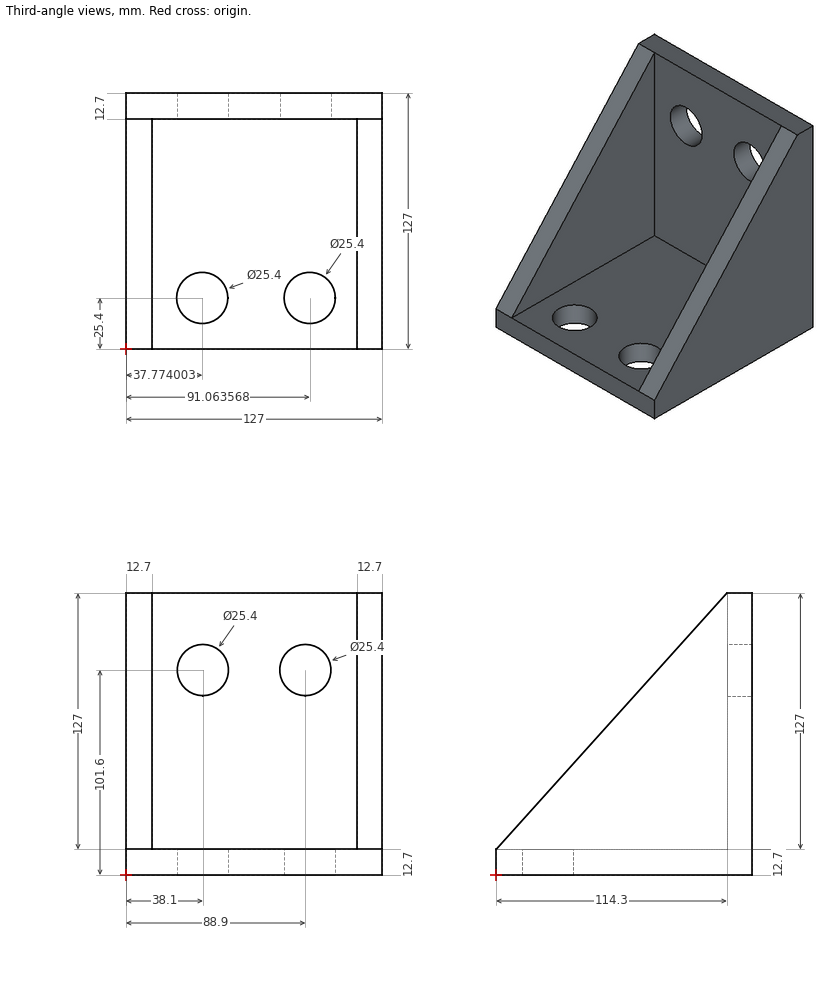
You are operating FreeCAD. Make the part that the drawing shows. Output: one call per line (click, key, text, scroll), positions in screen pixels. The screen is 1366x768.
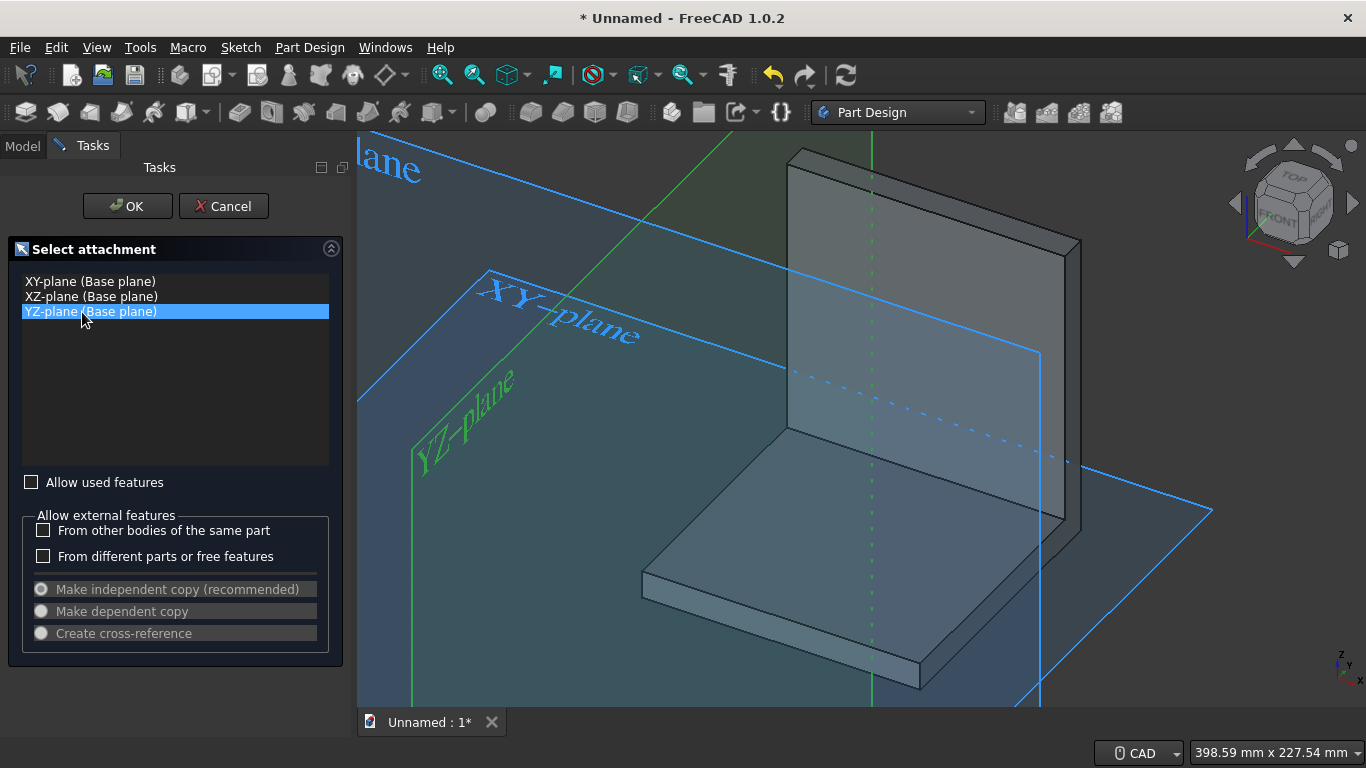
click(128, 206)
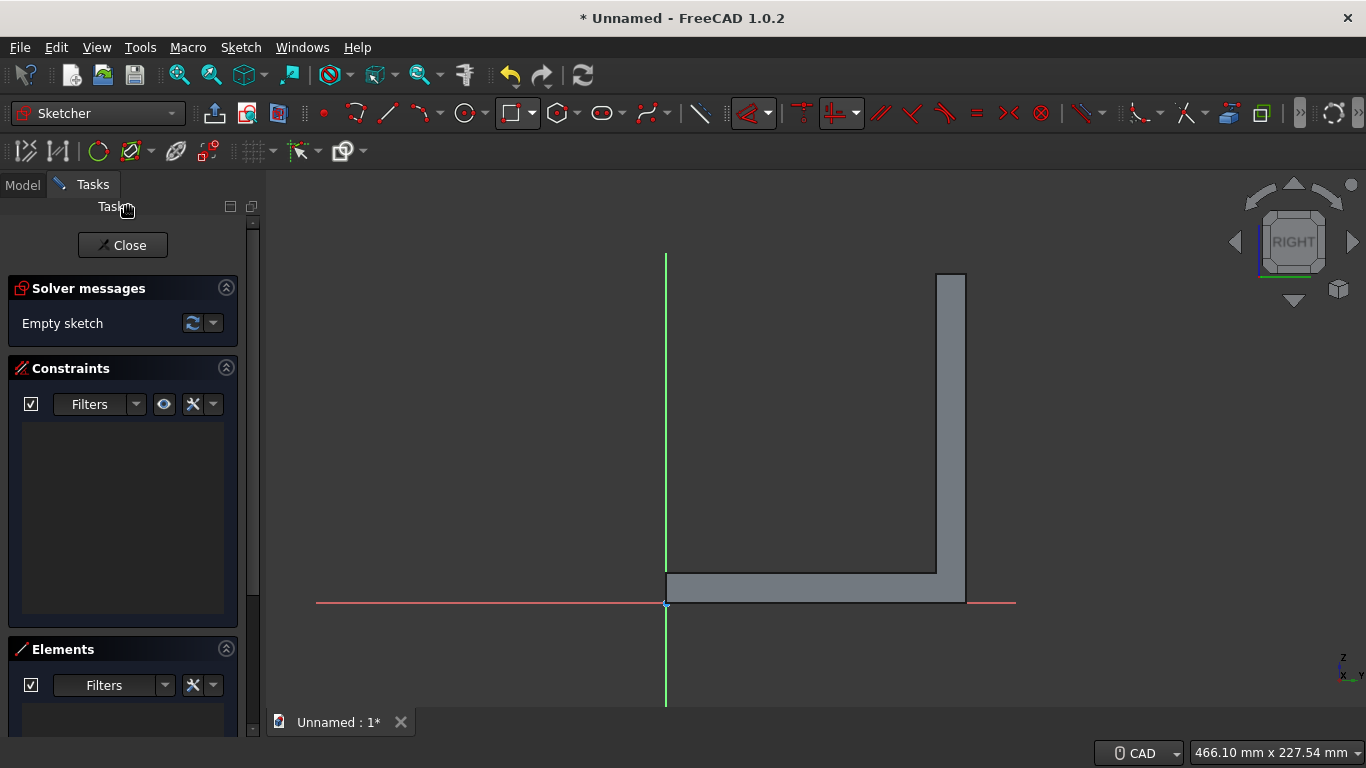
key(q)
key(s)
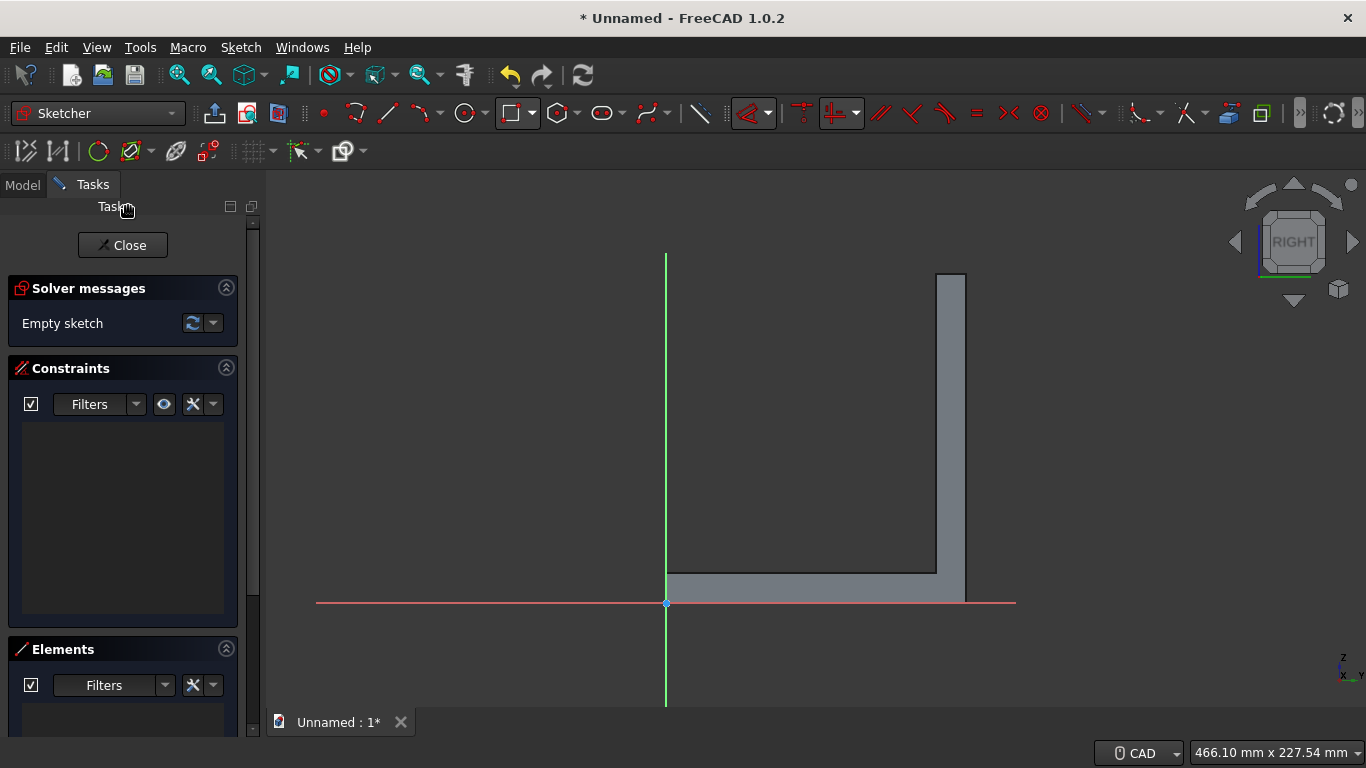
click(356, 114)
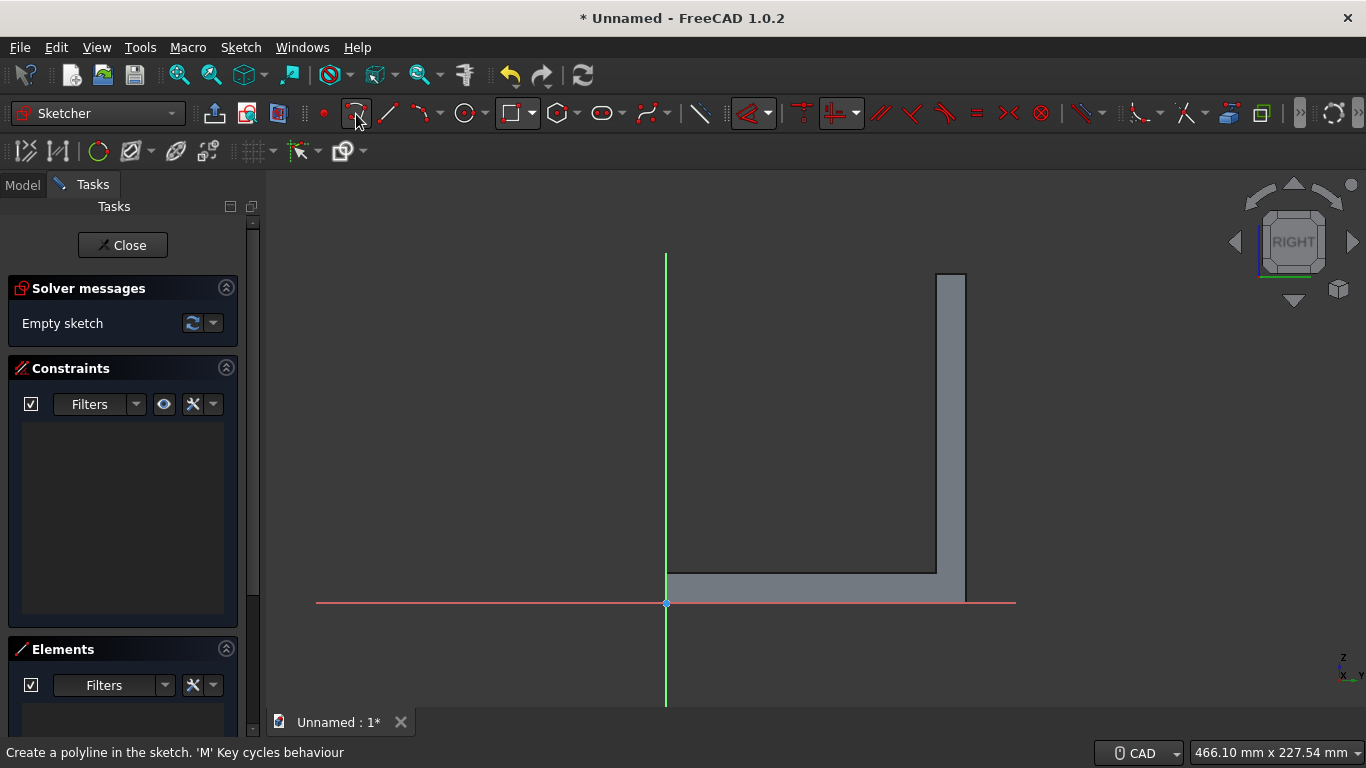
click(666, 573)
click(936, 274)
click(936, 573)
click(666, 574)
key(Escape)
key(Escape)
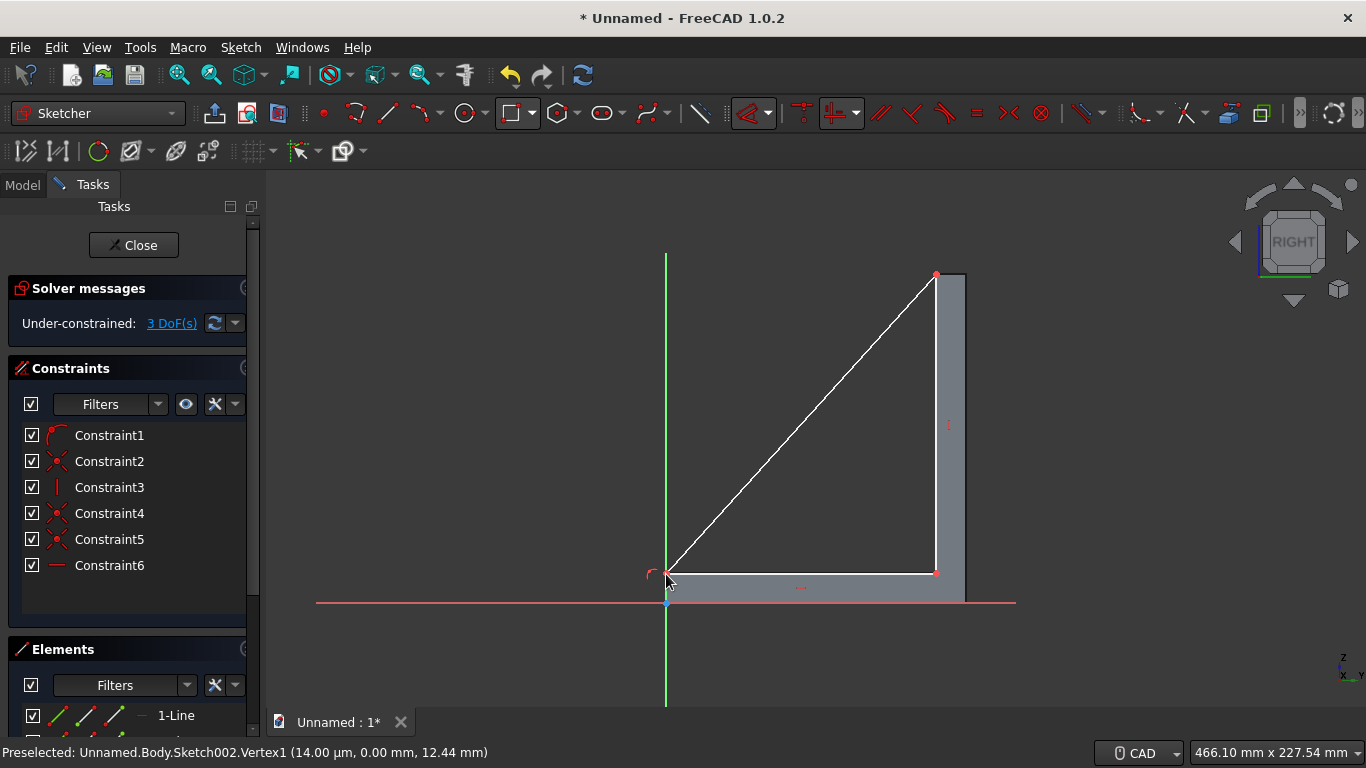
click(936, 365)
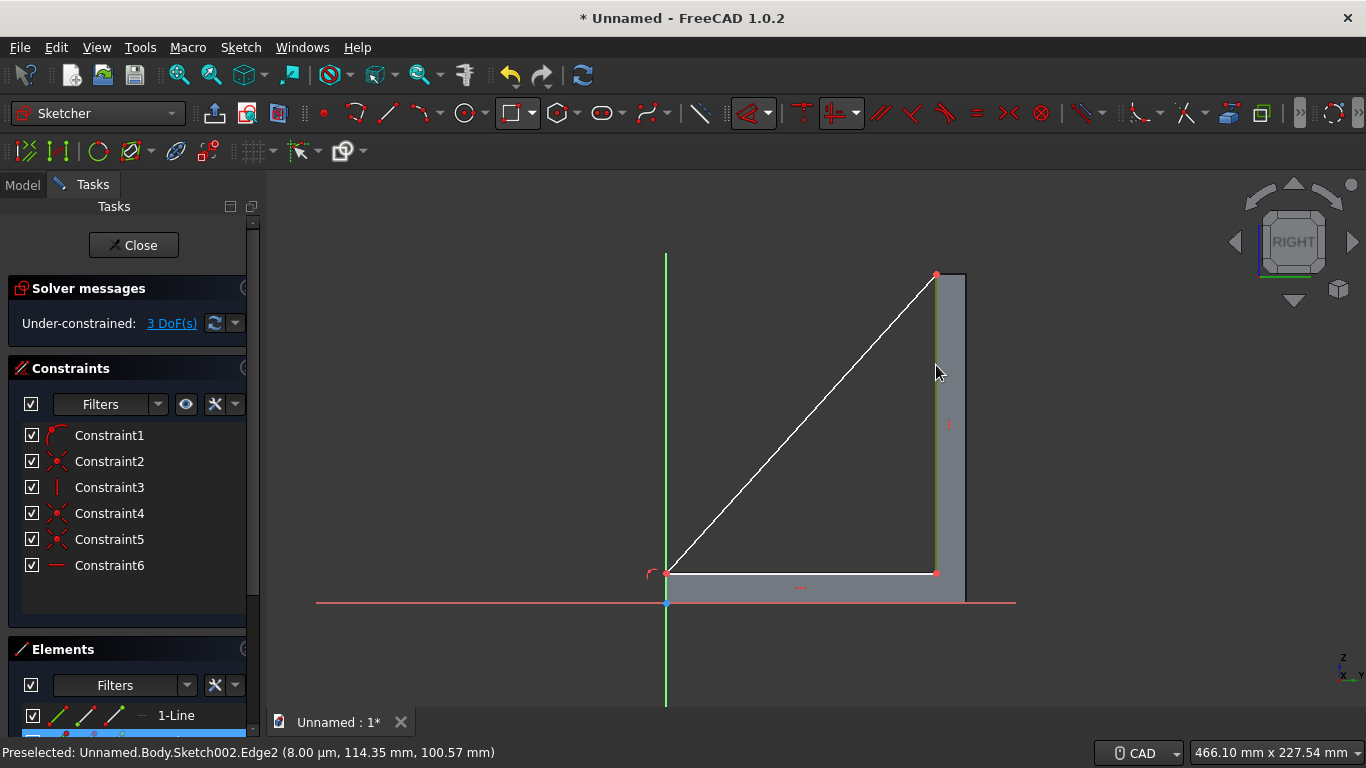
key(i)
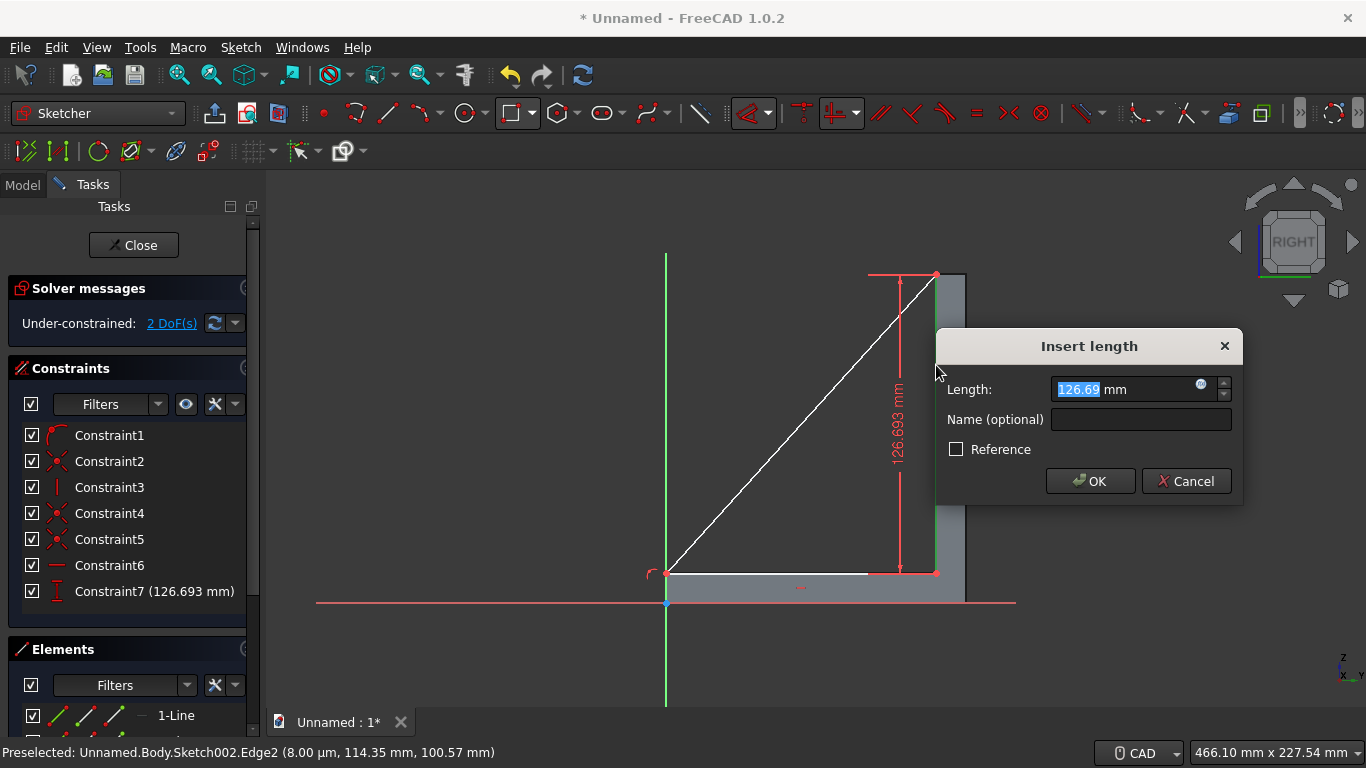
text(127)
key(Return)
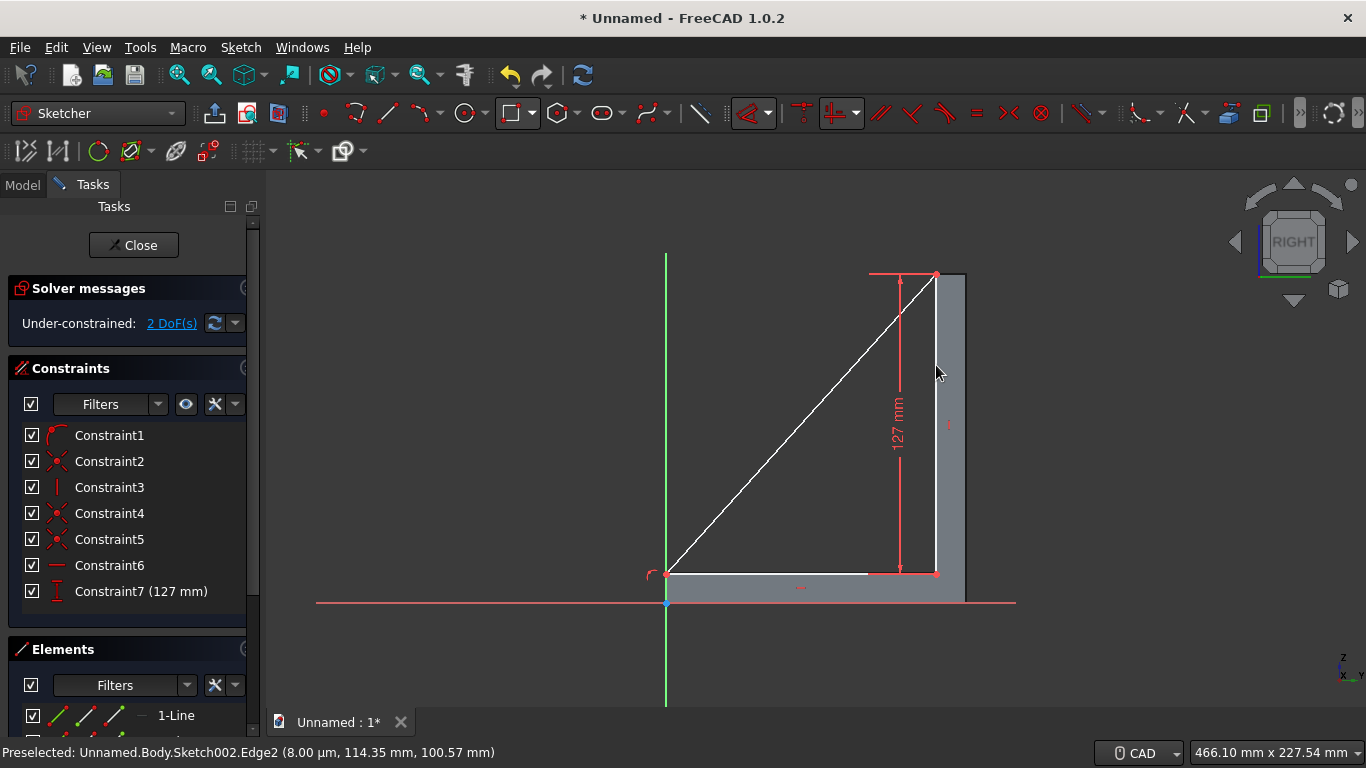
click(855, 574)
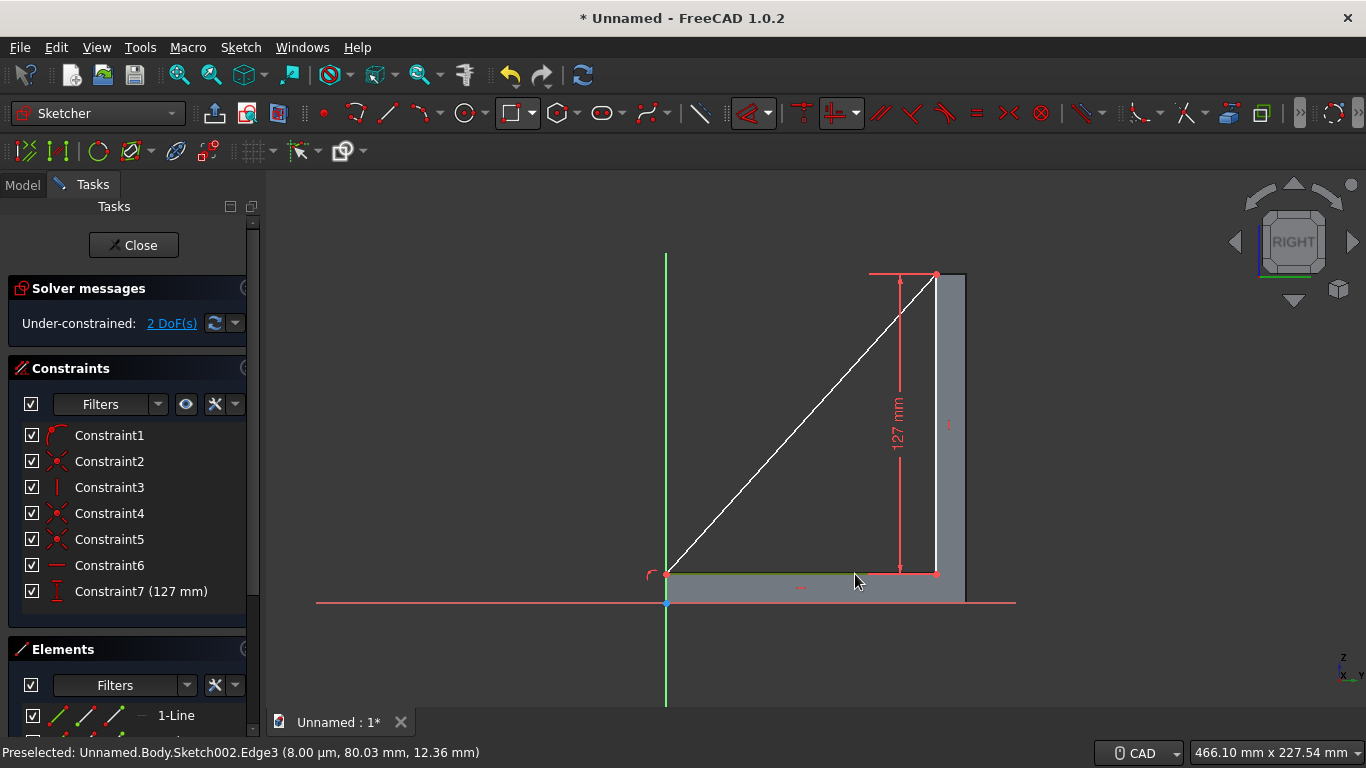
click(770, 114)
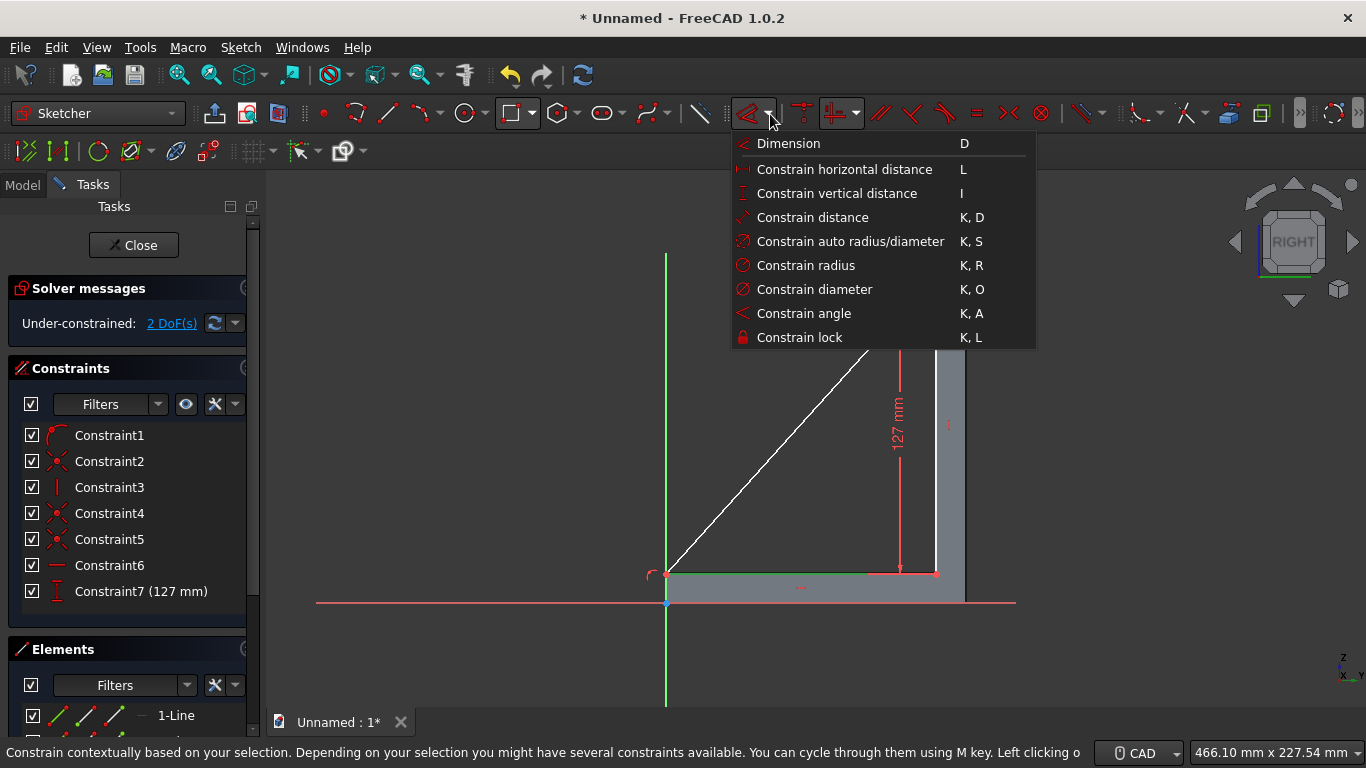
click(884, 169)